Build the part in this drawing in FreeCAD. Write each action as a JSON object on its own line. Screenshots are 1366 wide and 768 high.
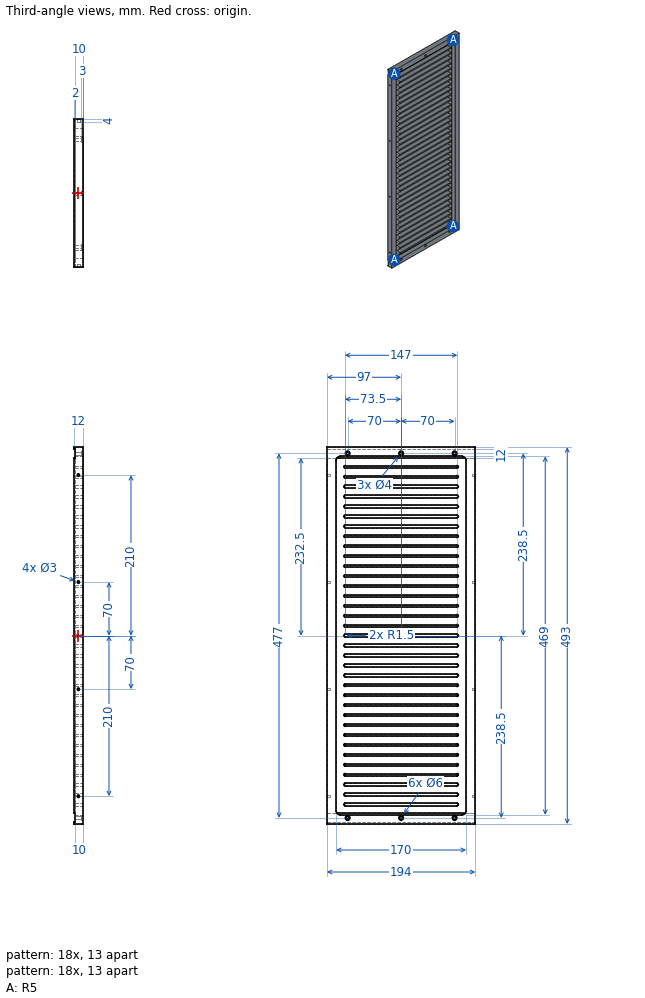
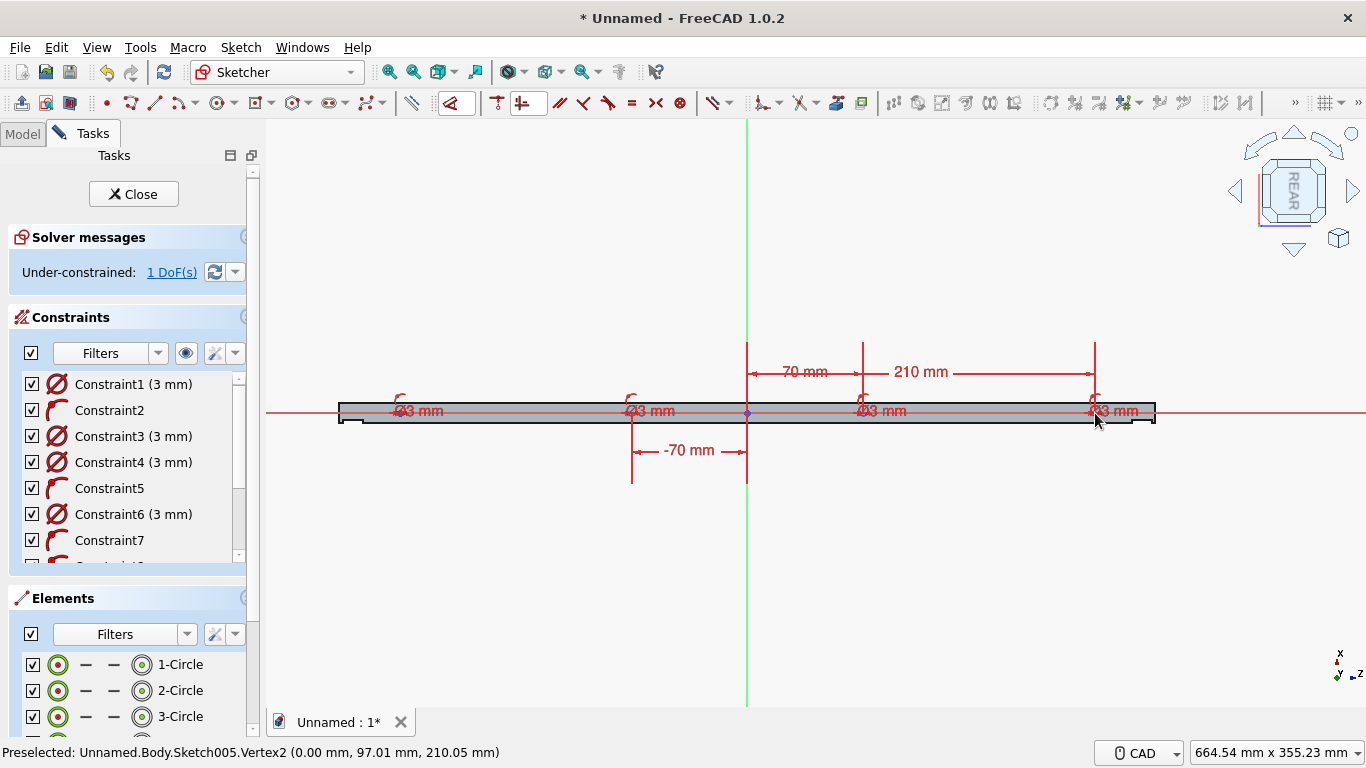
{"action": "left_click", "coordinate": [400, 413]}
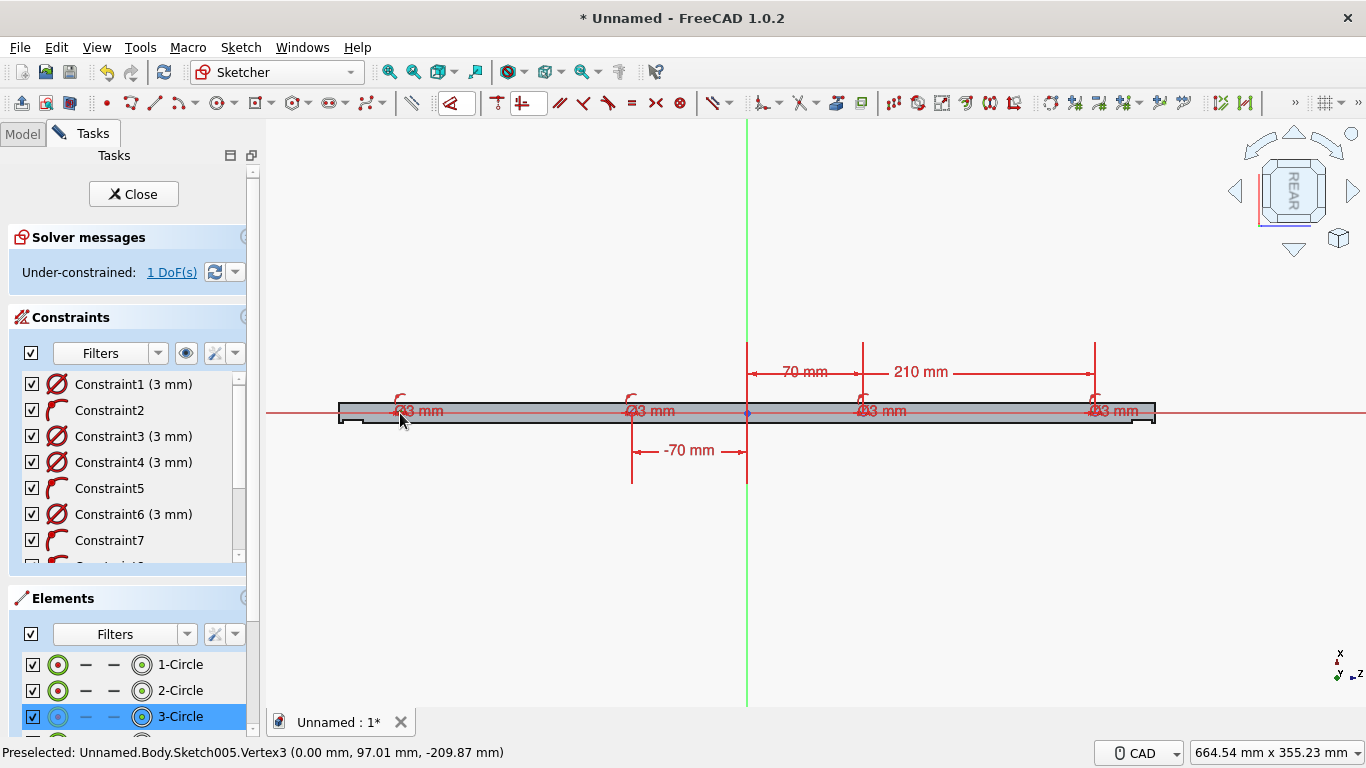
{"action": "left_click", "coordinate": [470, 104]}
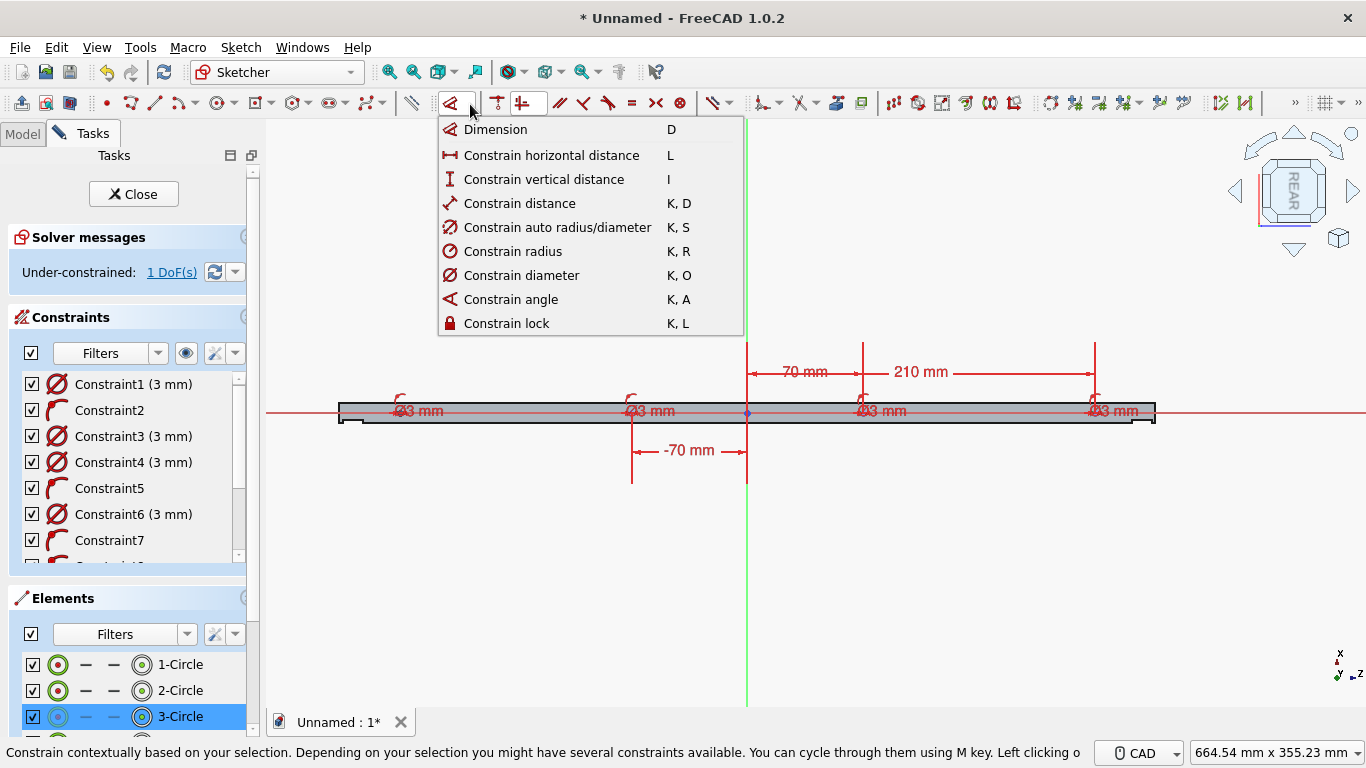
{"action": "left_click", "coordinate": [591, 155]}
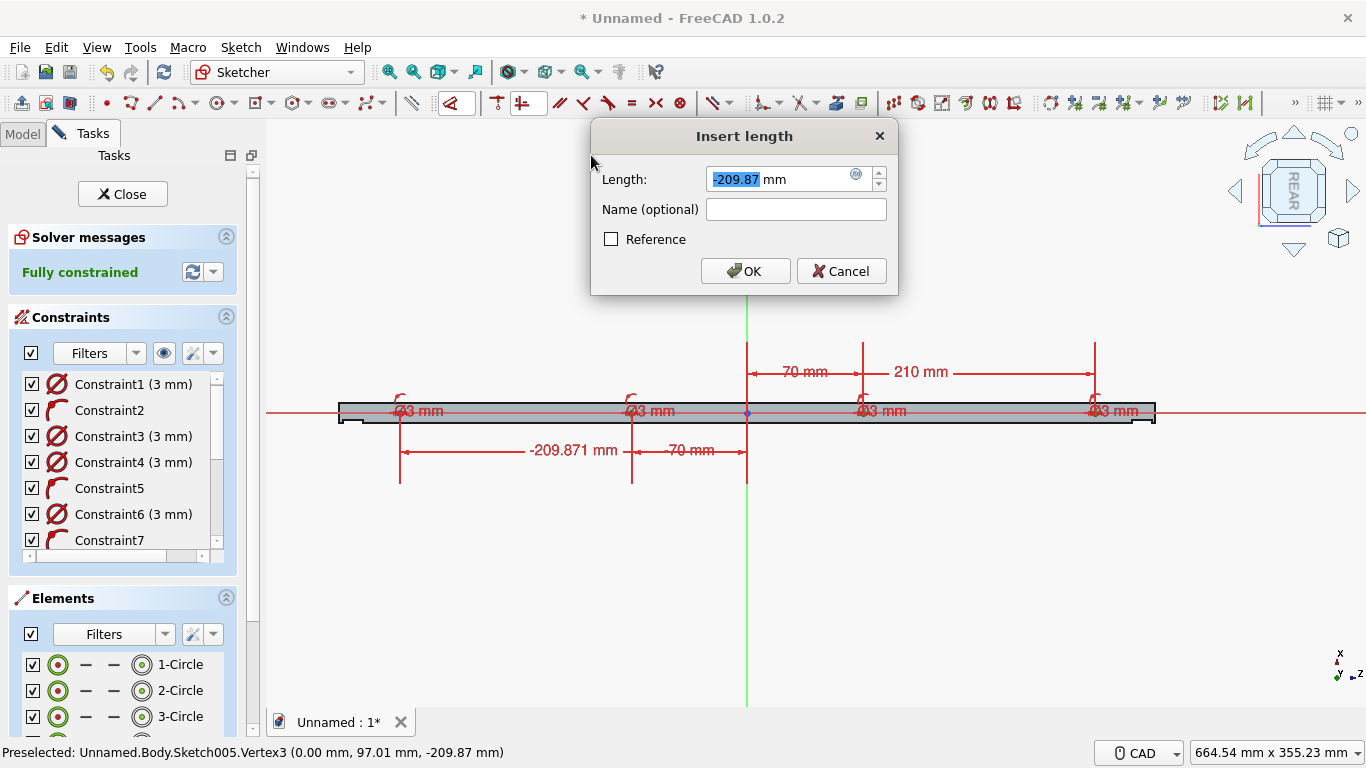
{"action": "type", "text": "-210"}
{"action": "key", "text": "Return"}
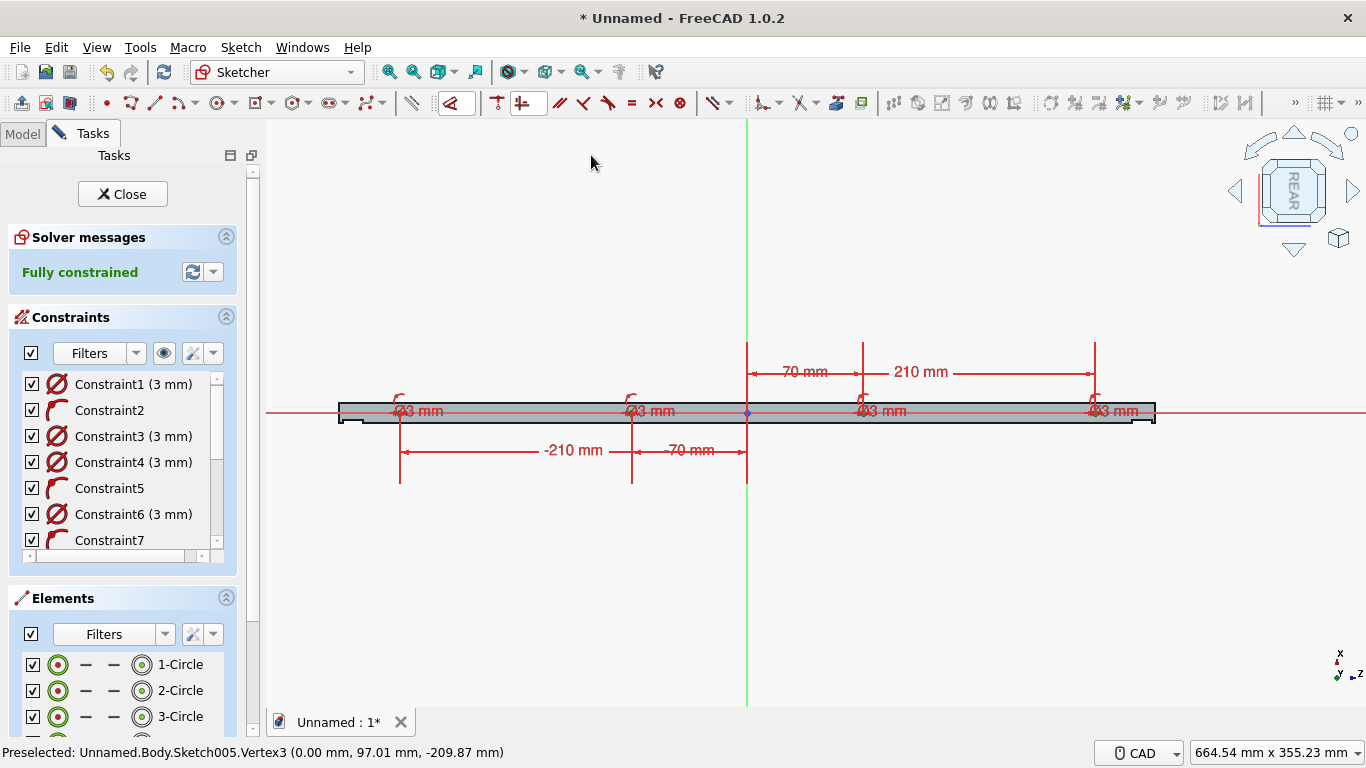
{"action": "left_click", "coordinate": [123, 194]}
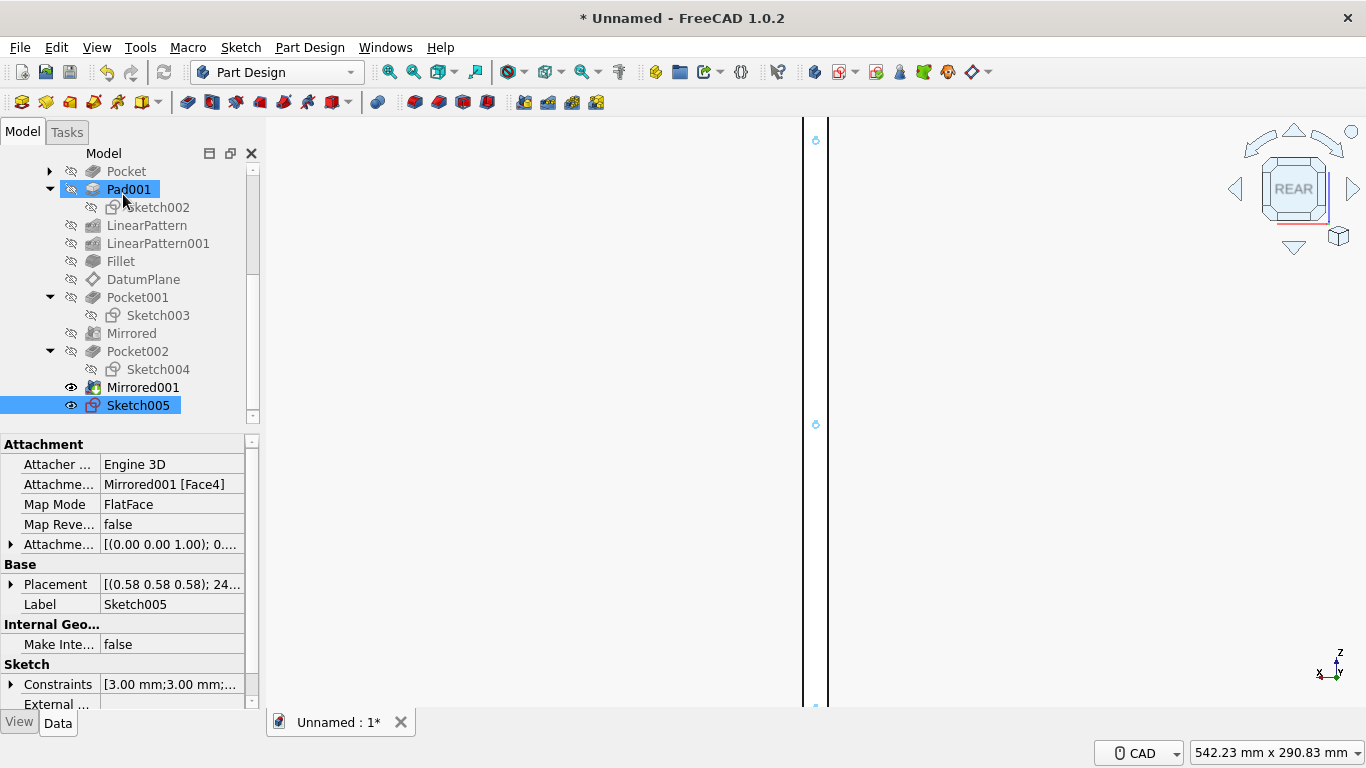
{"action": "left_click", "coordinate": [188, 102]}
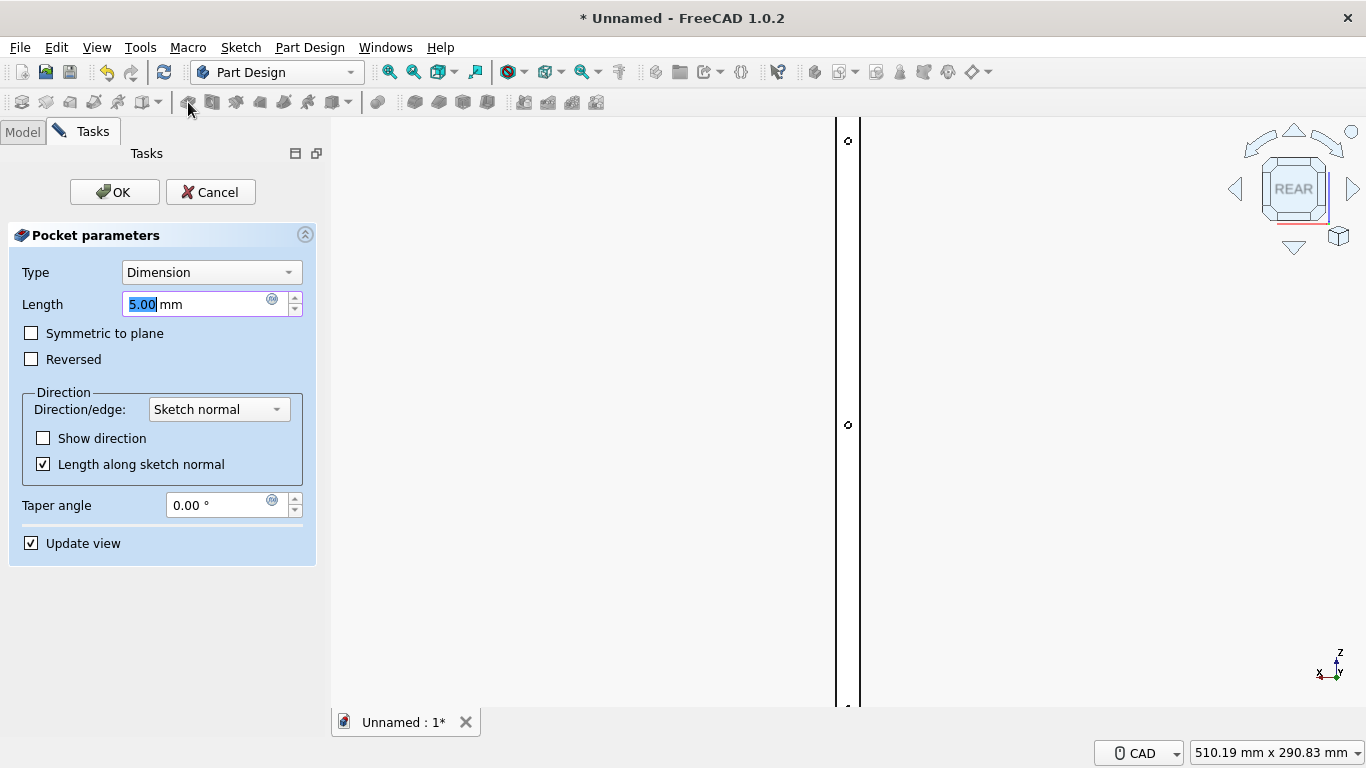
{"action": "type", "text": "4"}
{"action": "key", "text": "Tab"}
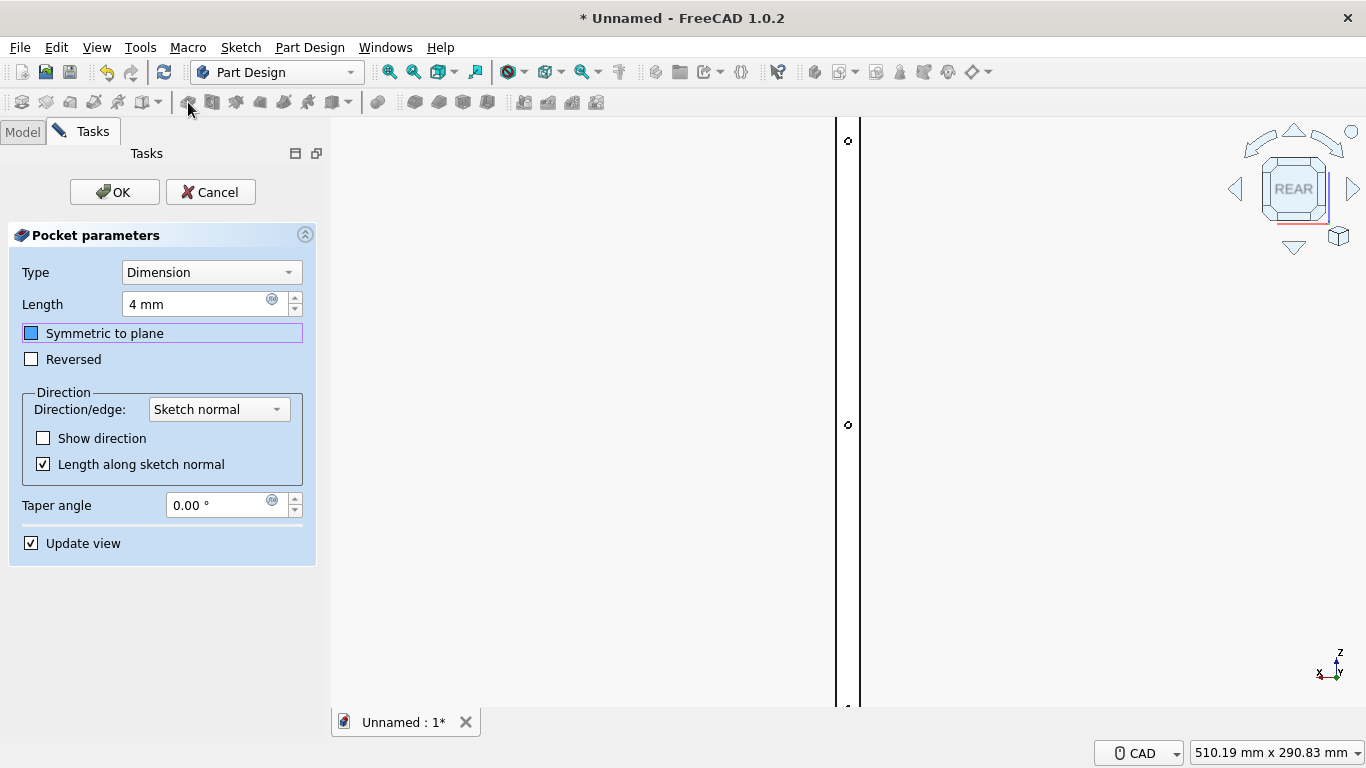
{"action": "left_click", "coordinate": [115, 192]}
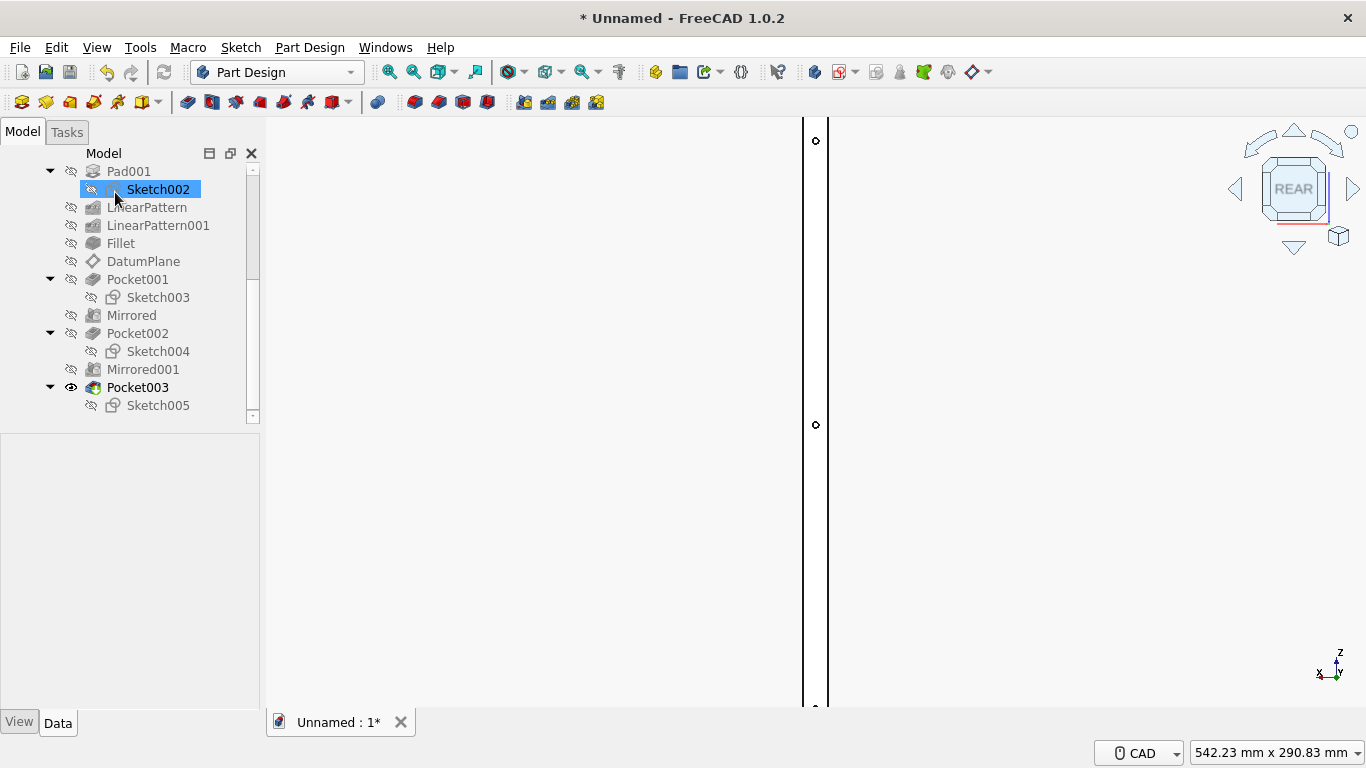
{"action": "key", "text": "v f"}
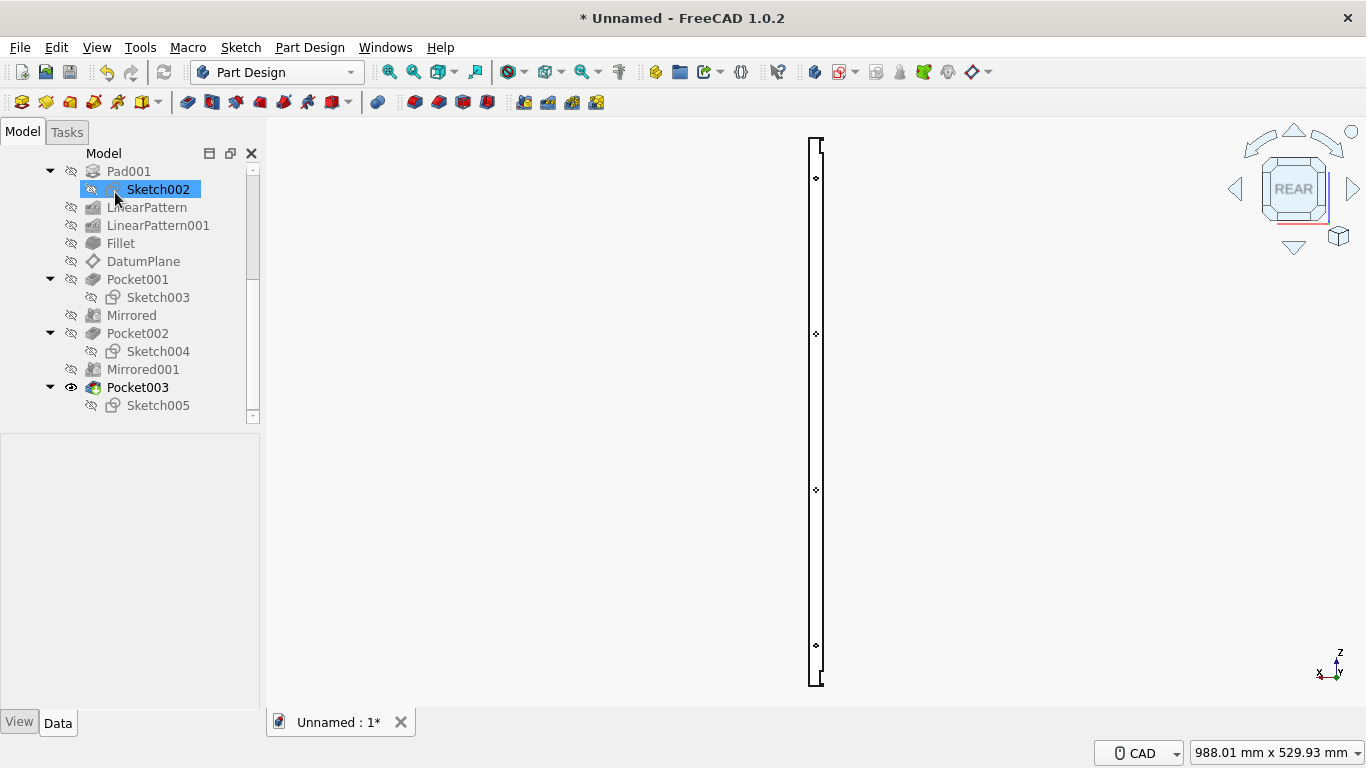
{"action": "left_click", "coordinate": [116, 387]}